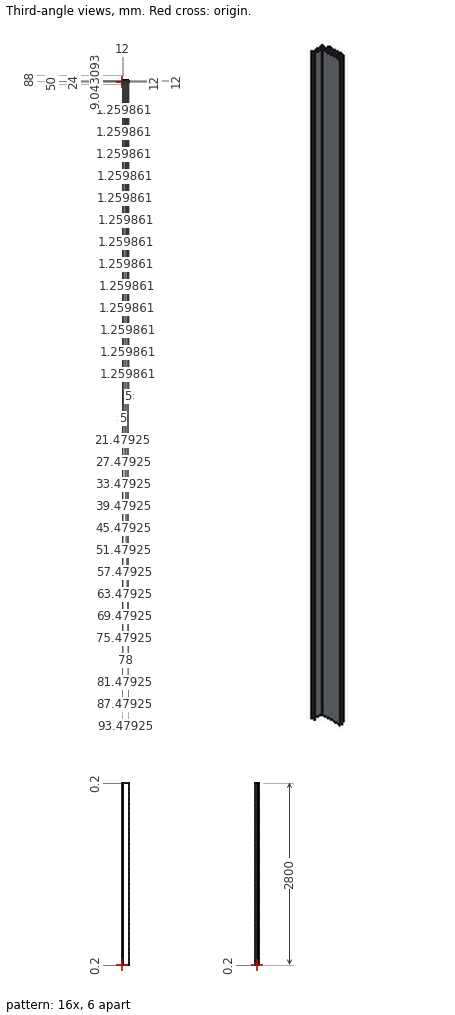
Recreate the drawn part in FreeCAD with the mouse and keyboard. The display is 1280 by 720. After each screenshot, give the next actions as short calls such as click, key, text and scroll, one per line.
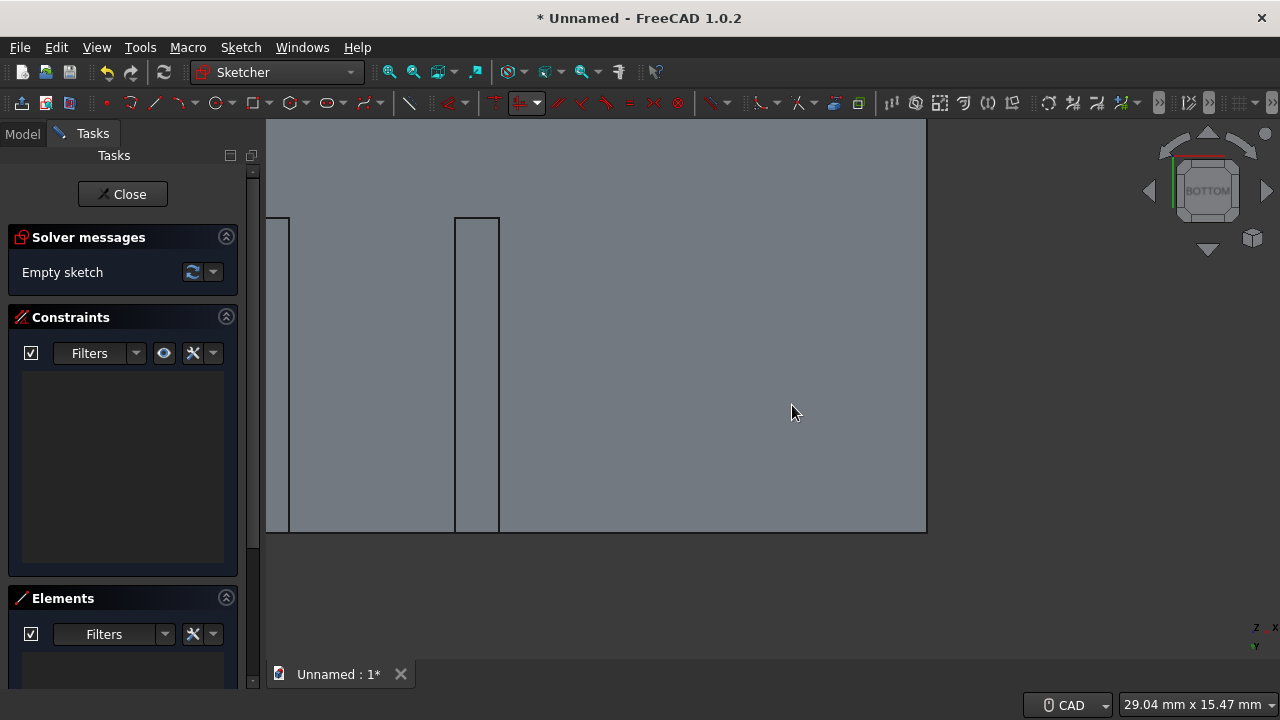
click(254, 104)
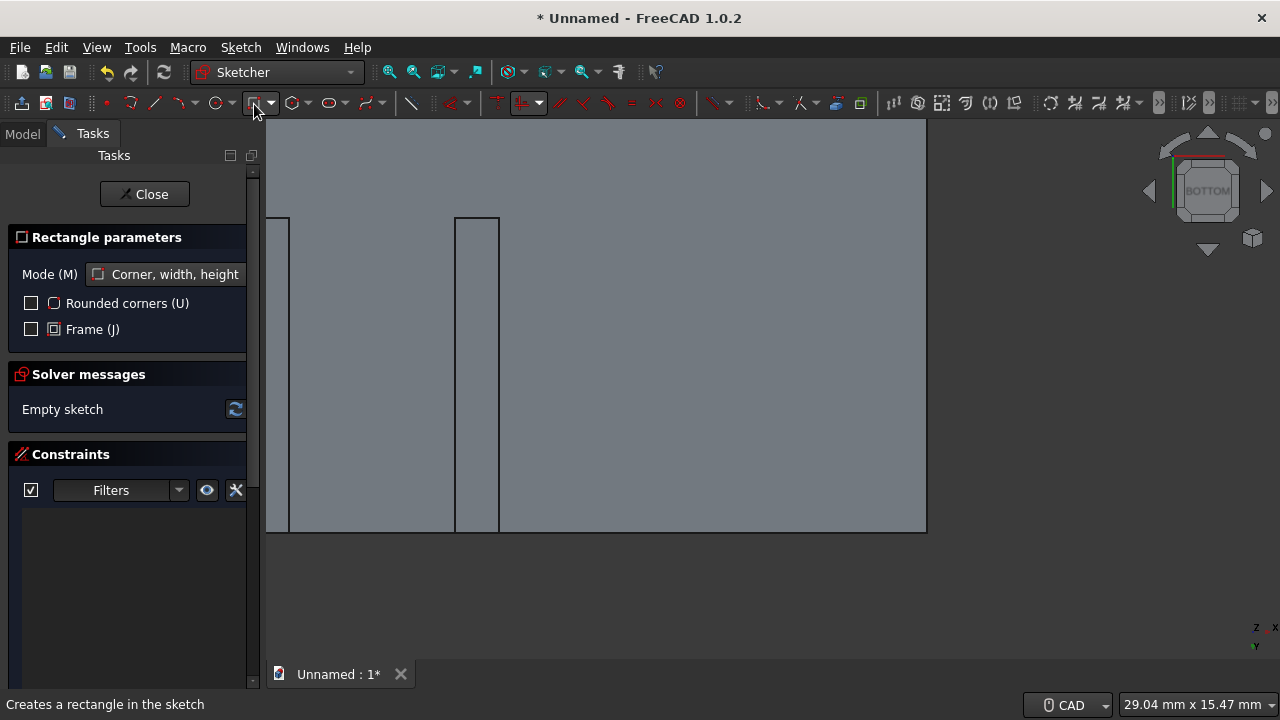
click(664, 218)
move(708, 533)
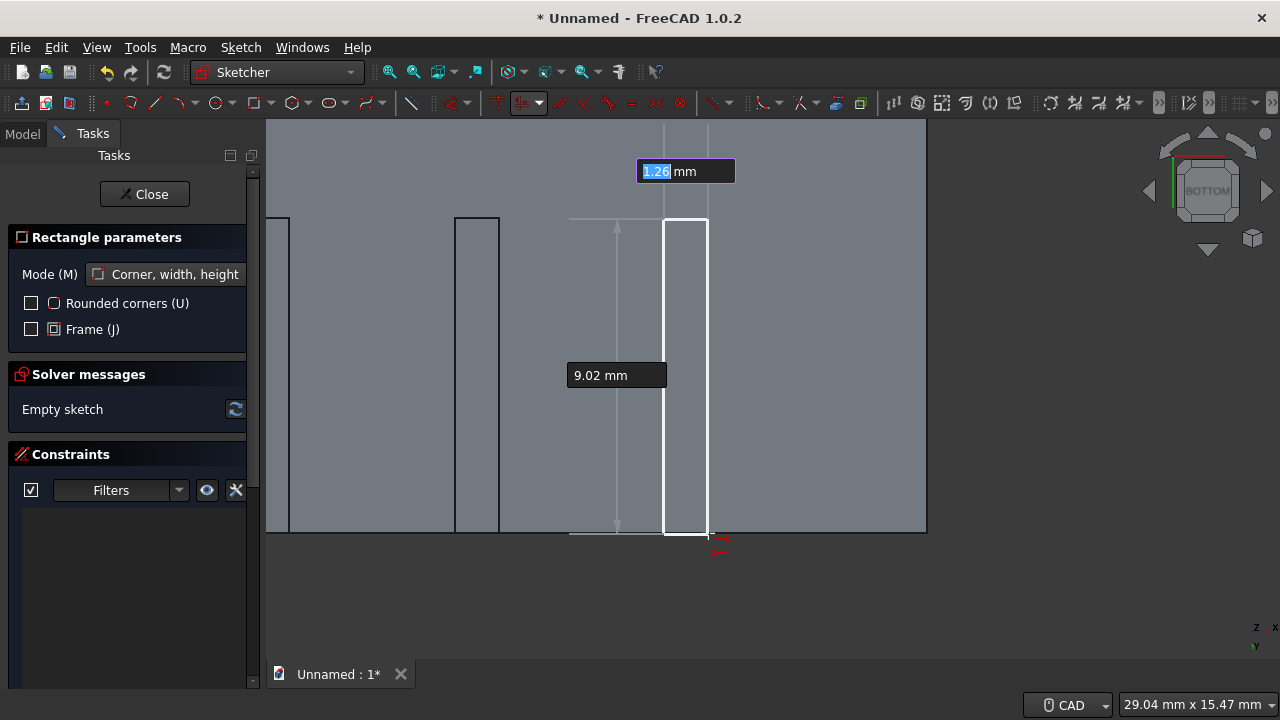
text(1.259861)
key(Tab)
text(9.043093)
key(Return)
key(Escape)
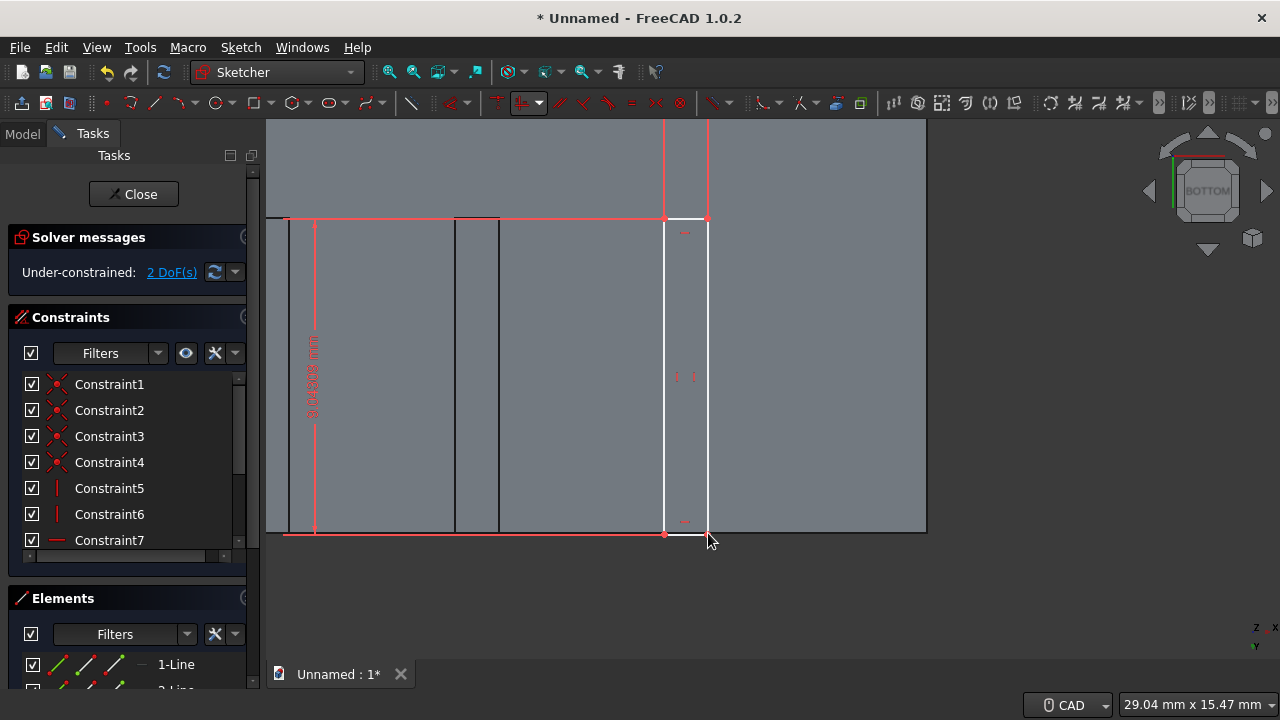
click(450, 104)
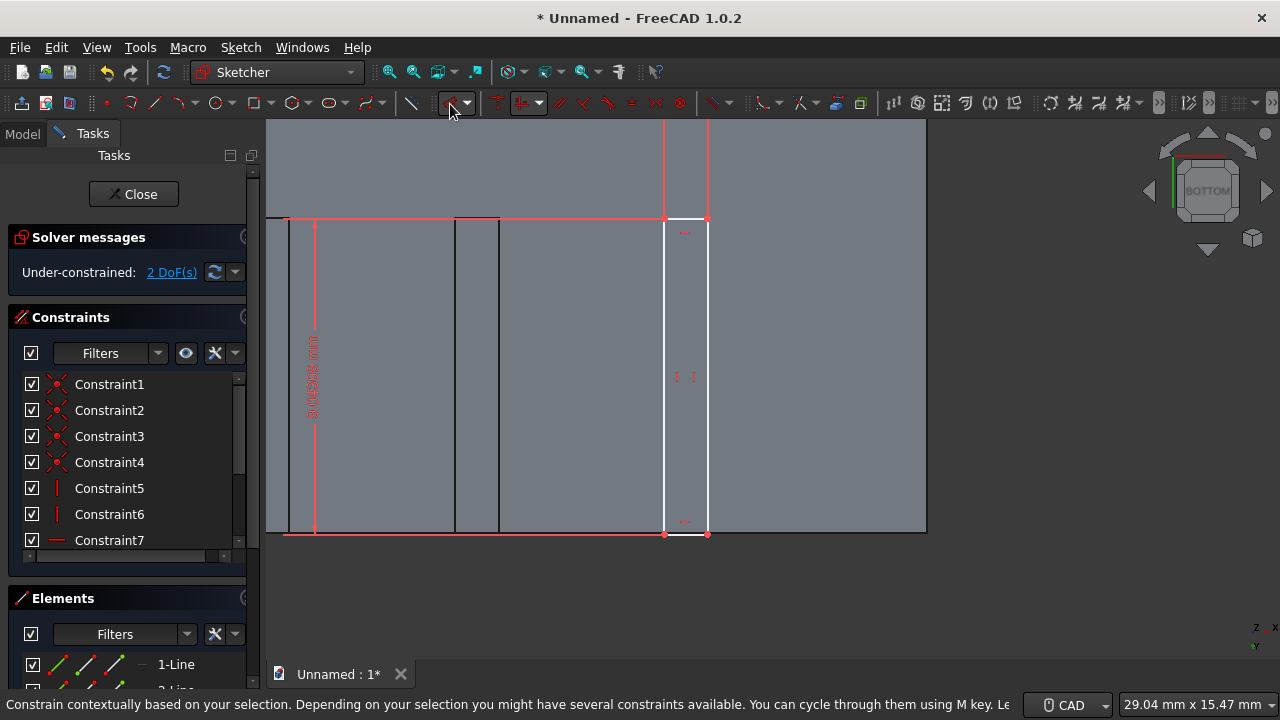
click(664, 535)
click(698, 205)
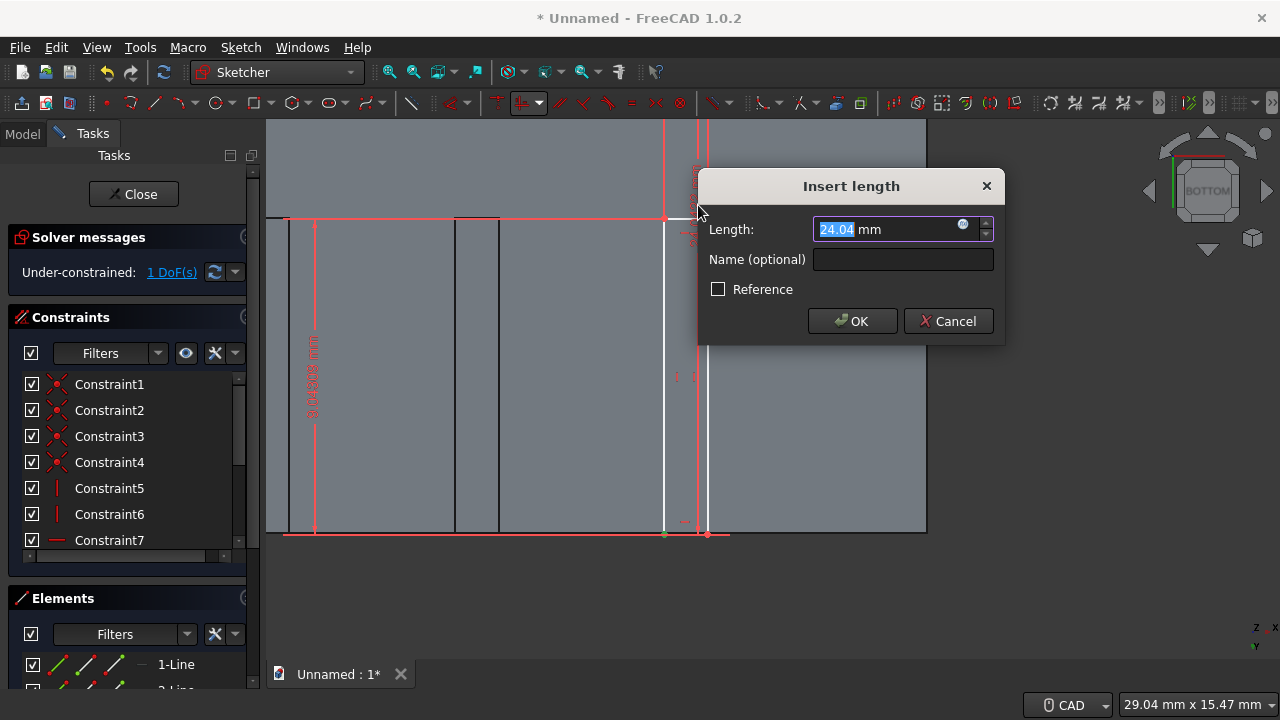
text(24)
key(Return)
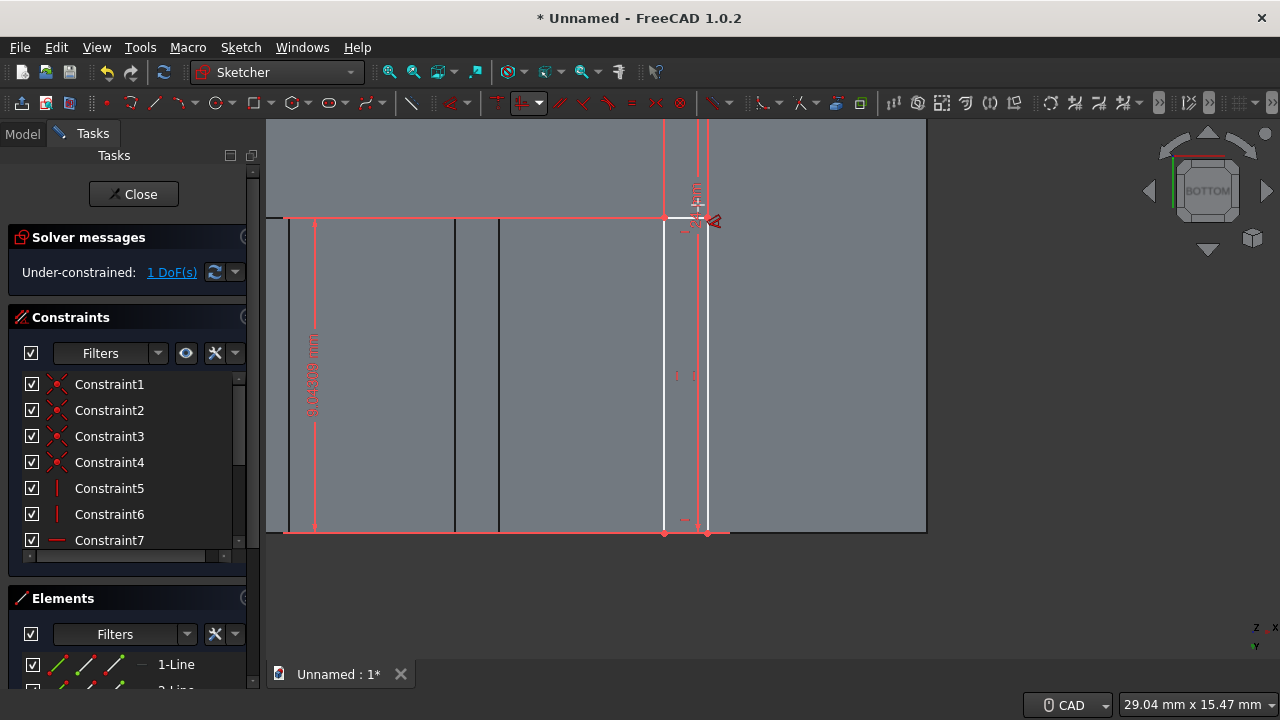
click(664, 218)
click(479, 252)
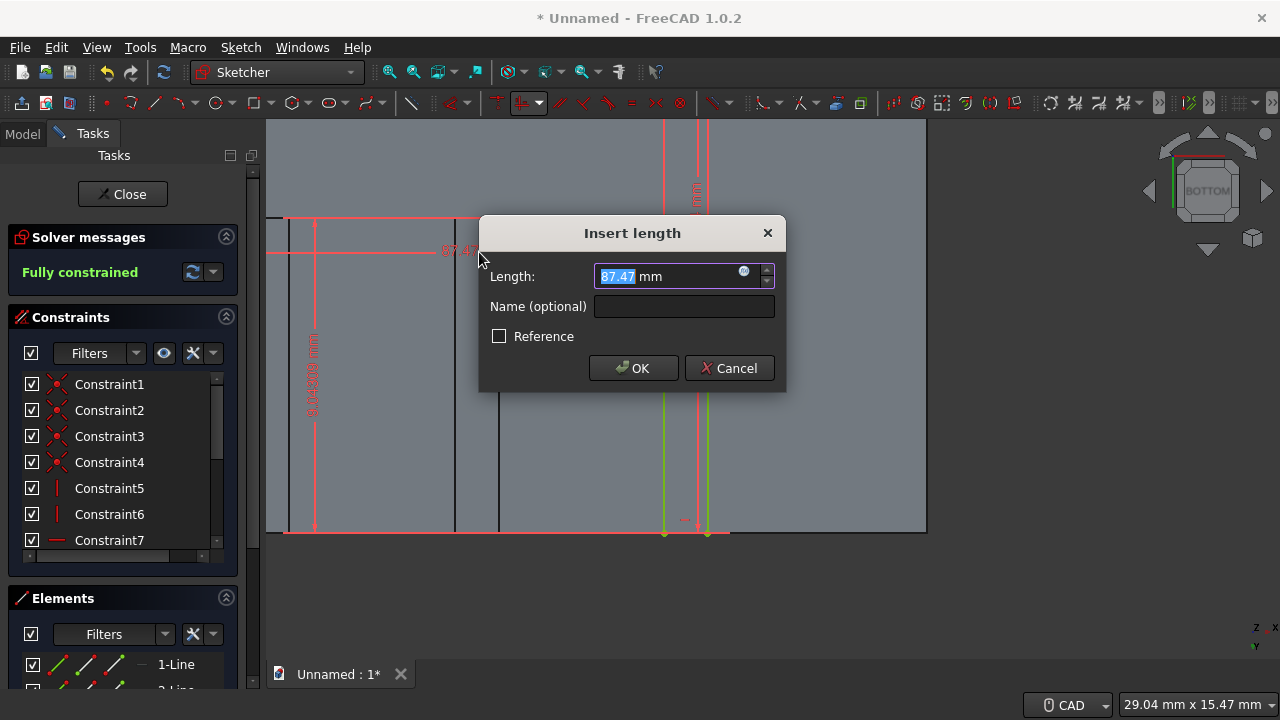
text(87.47925)
key(Return)
key(Escape)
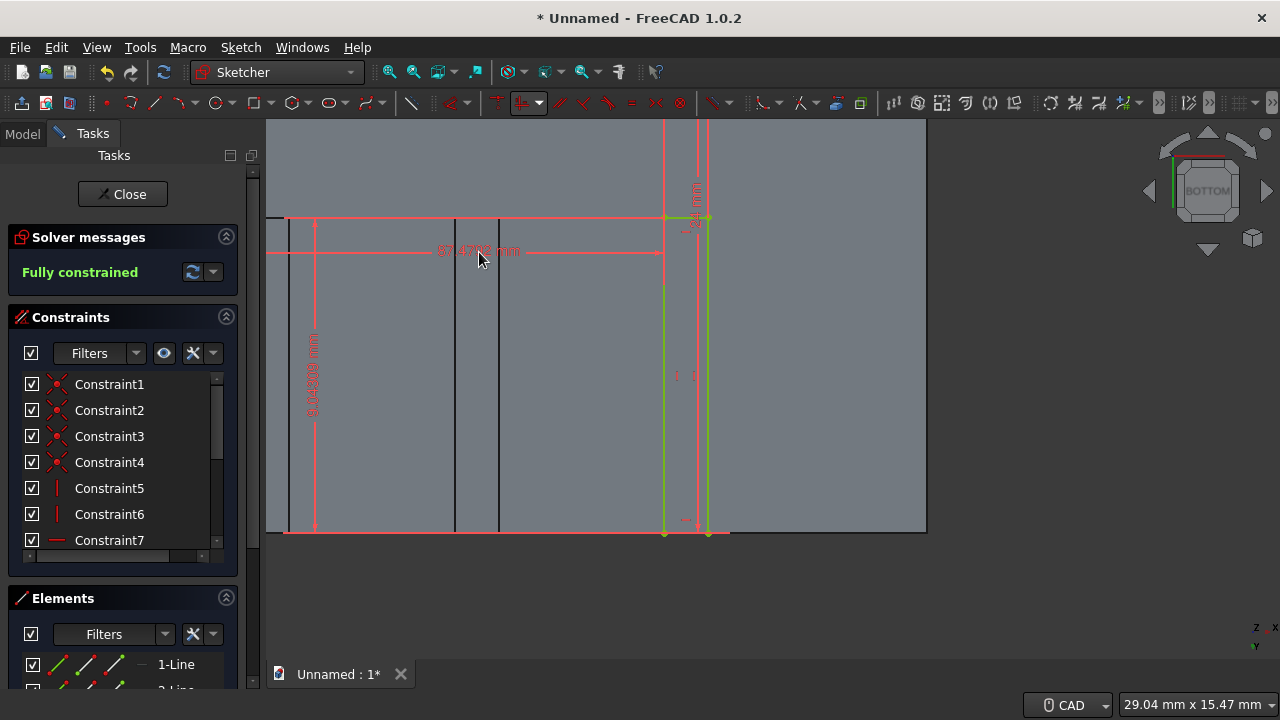
click(123, 194)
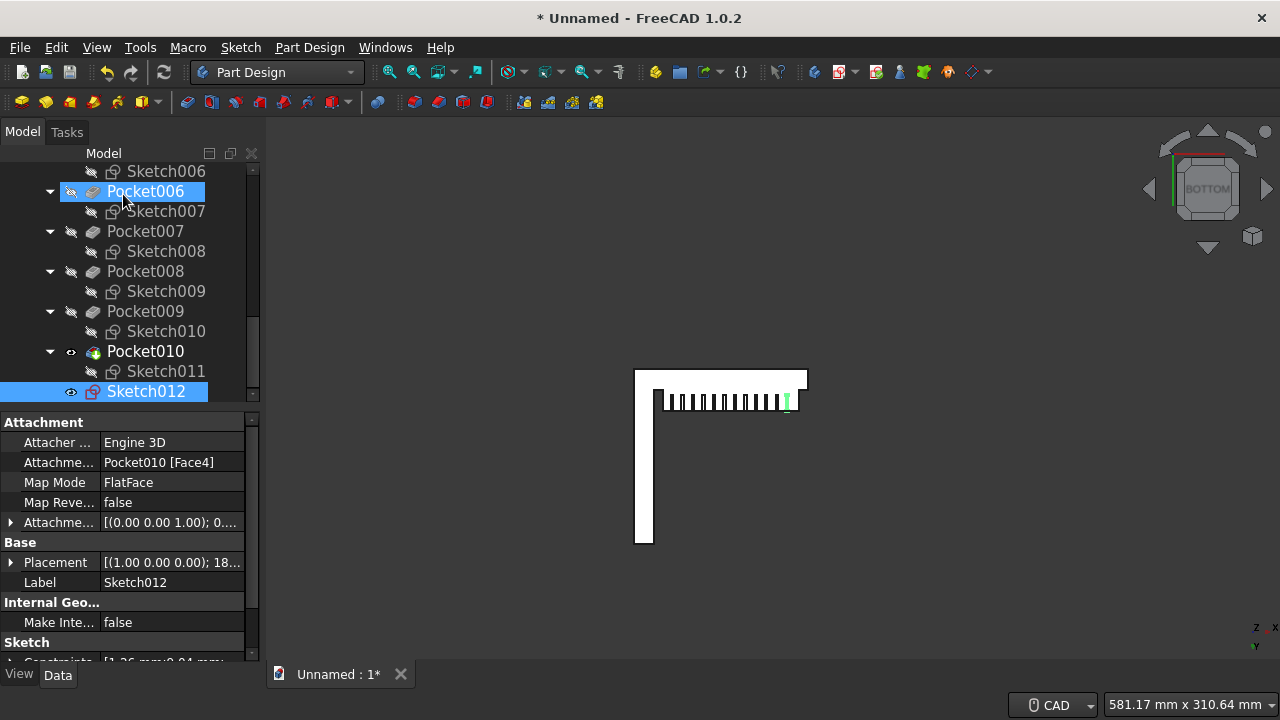
click(188, 102)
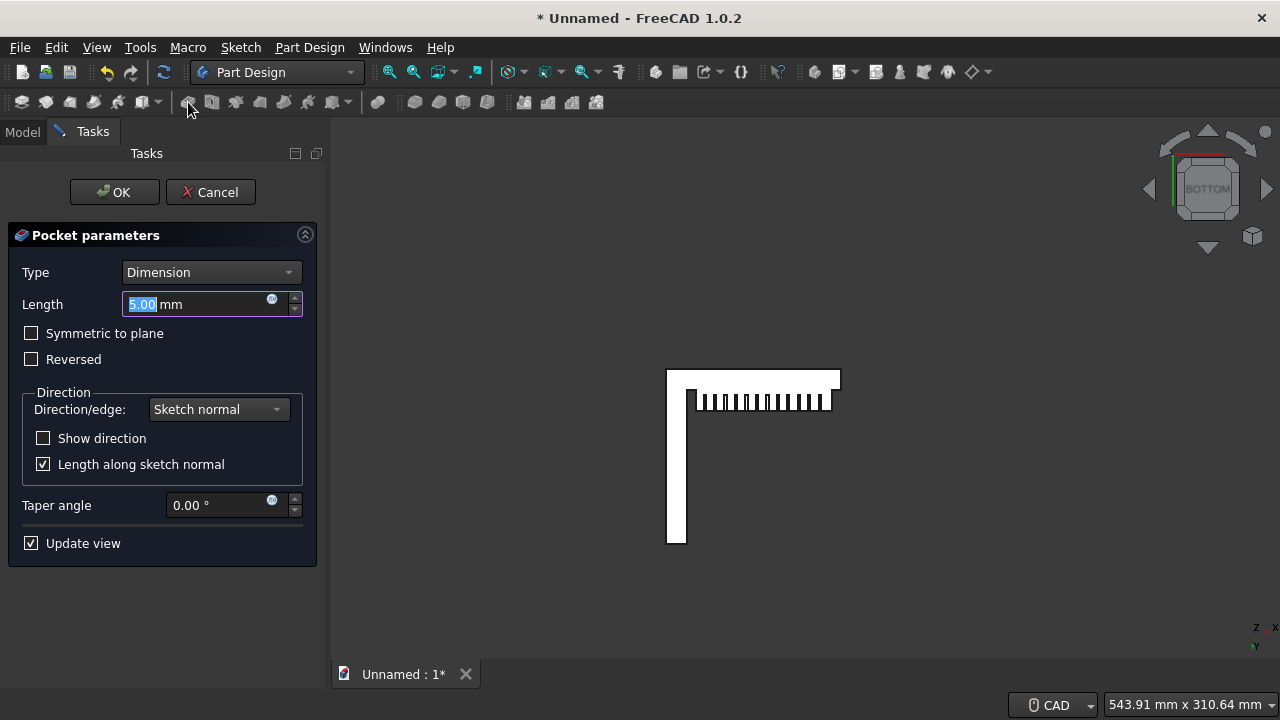
text(0.2)
key(Tab)